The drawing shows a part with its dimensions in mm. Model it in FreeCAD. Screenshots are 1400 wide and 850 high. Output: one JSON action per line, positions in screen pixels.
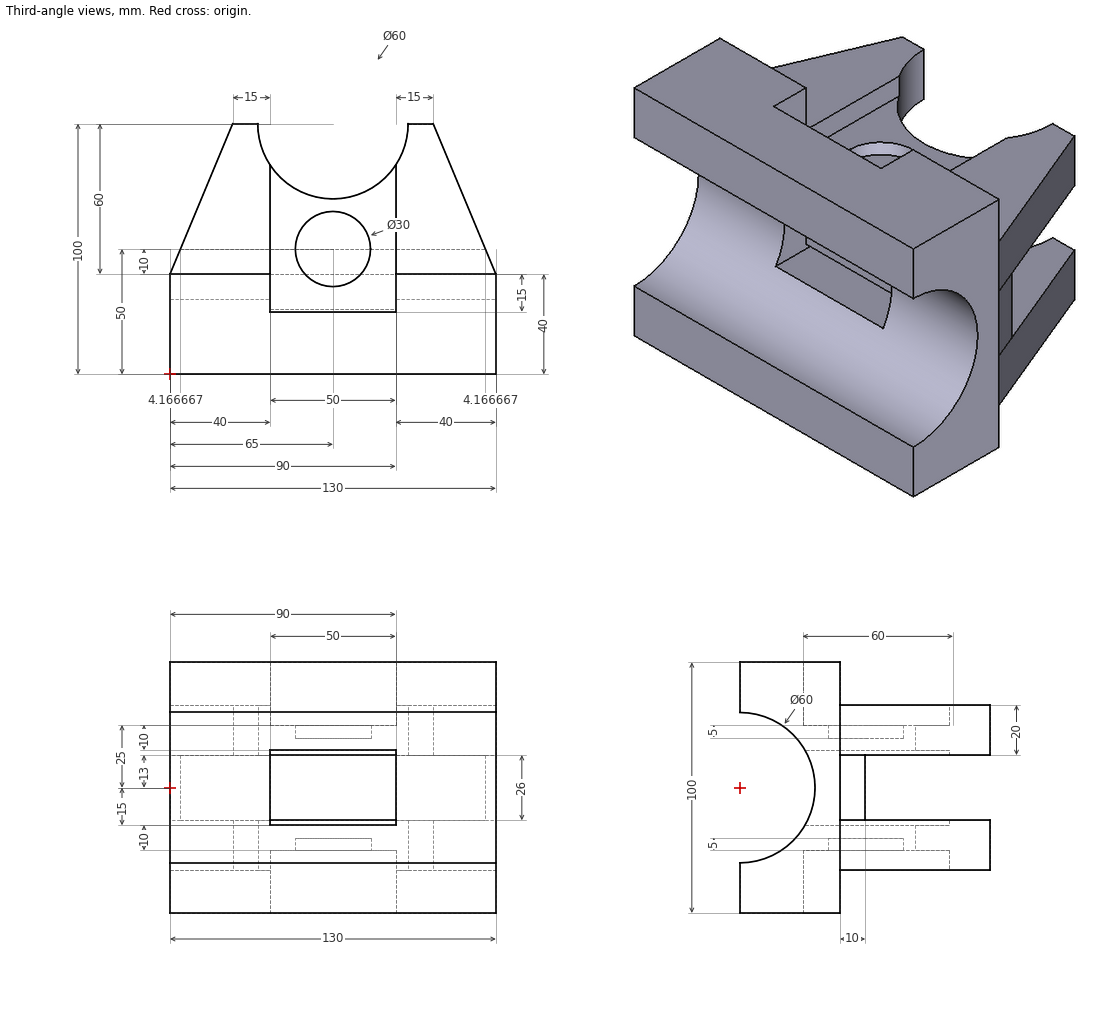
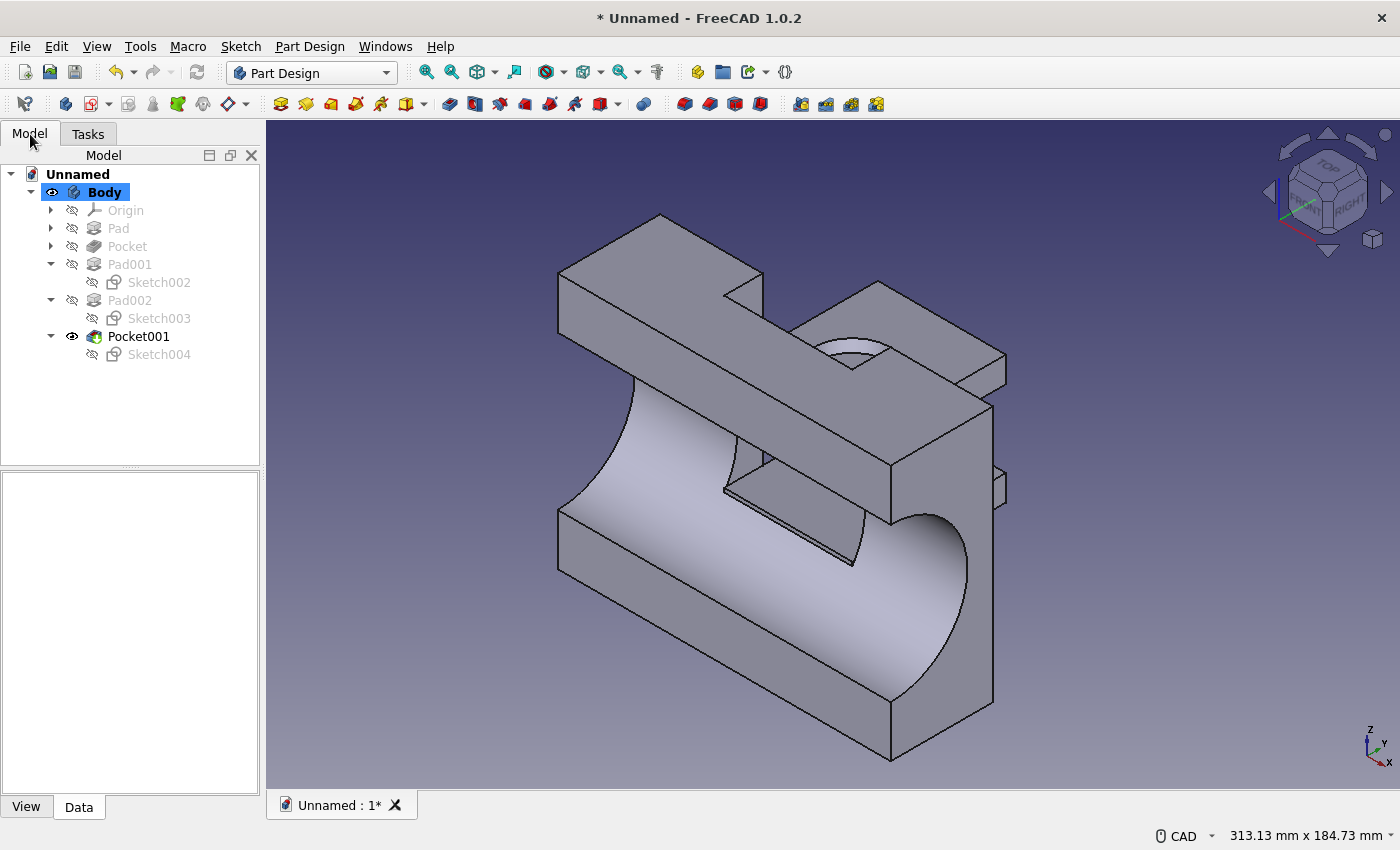
{"action": "left_click", "coordinate": [51, 210]}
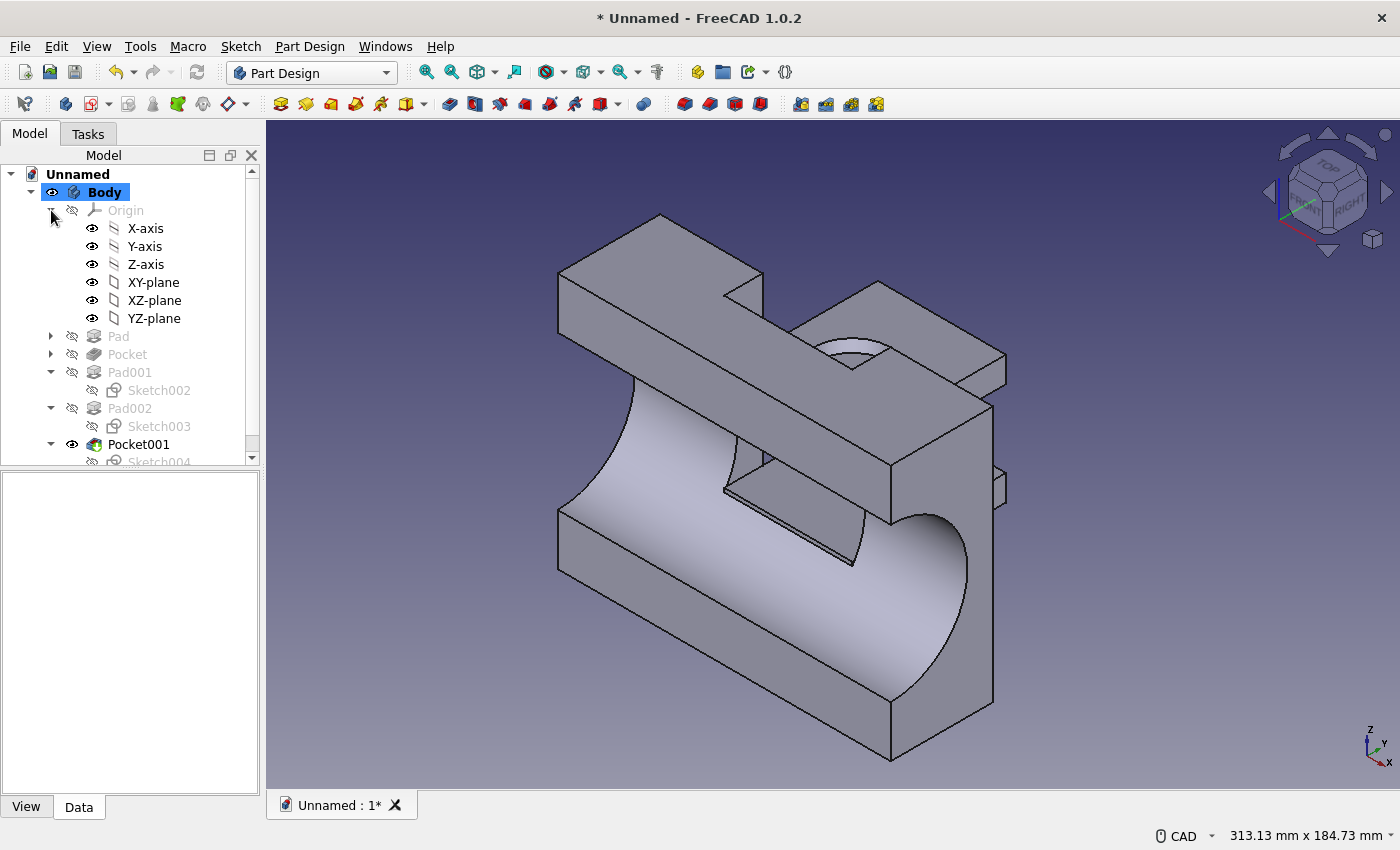
{"action": "left_click", "coordinate": [137, 282]}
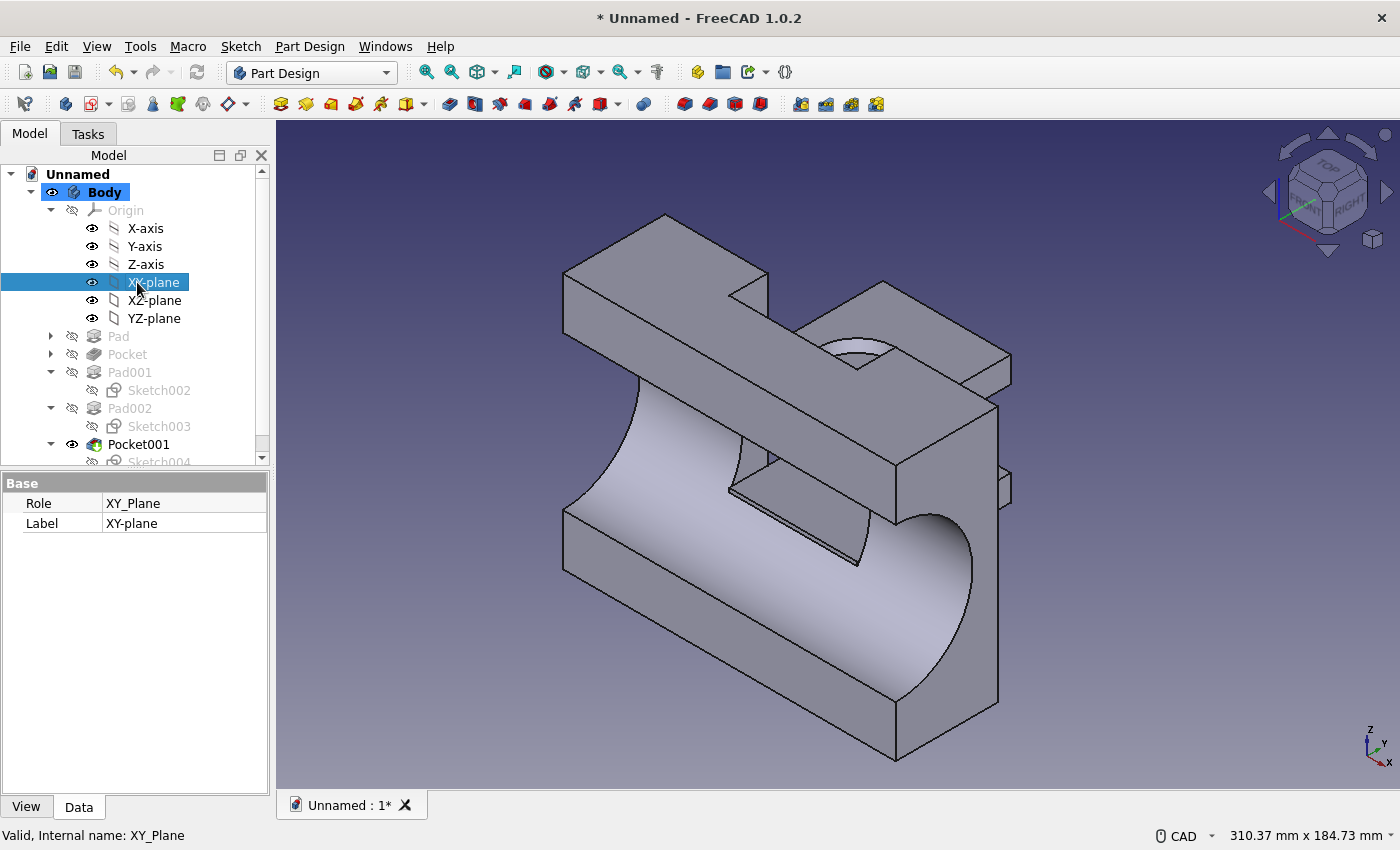
{"action": "left_click", "coordinate": [228, 104]}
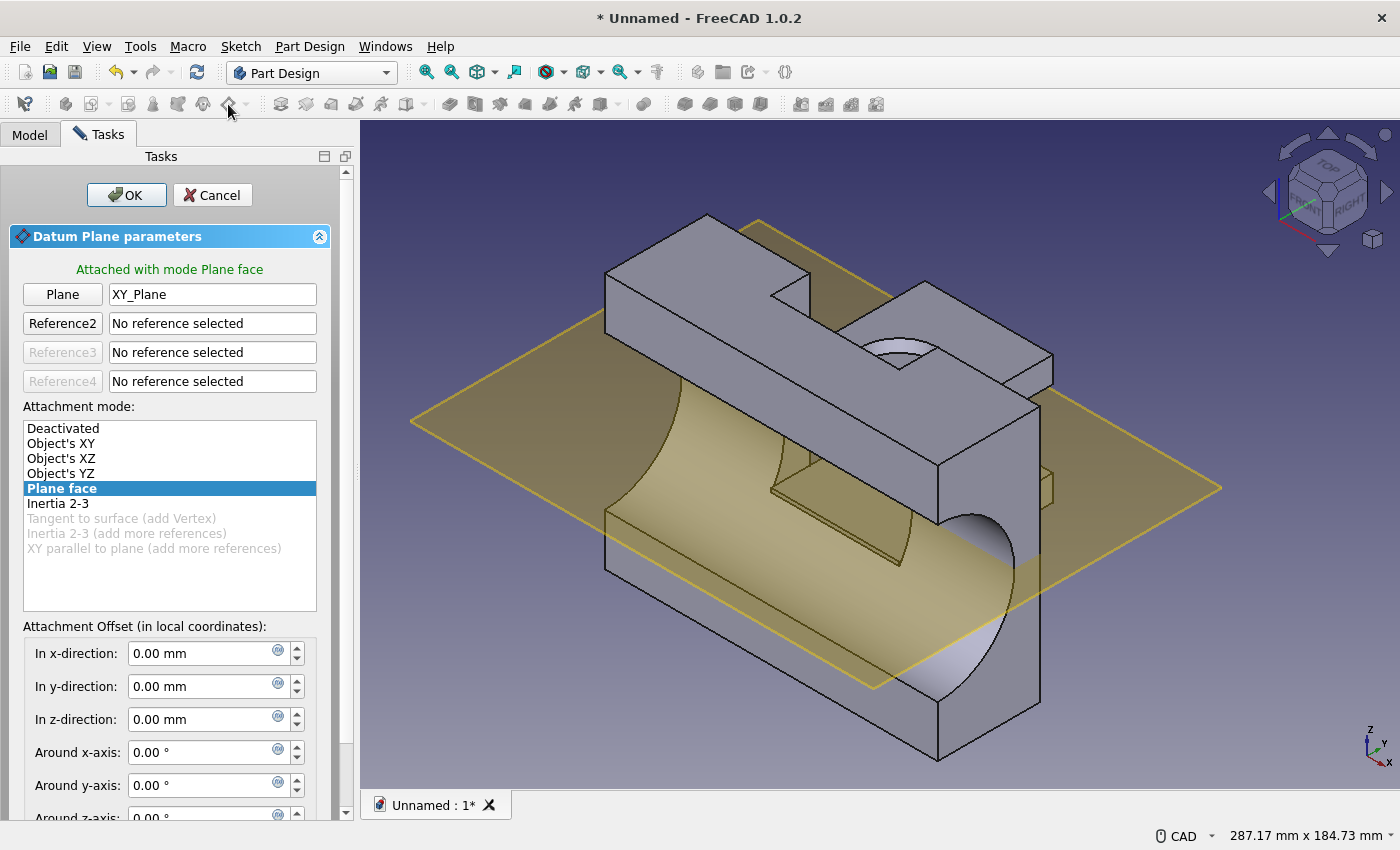
{"action": "triple_click", "coordinate": [210, 720]}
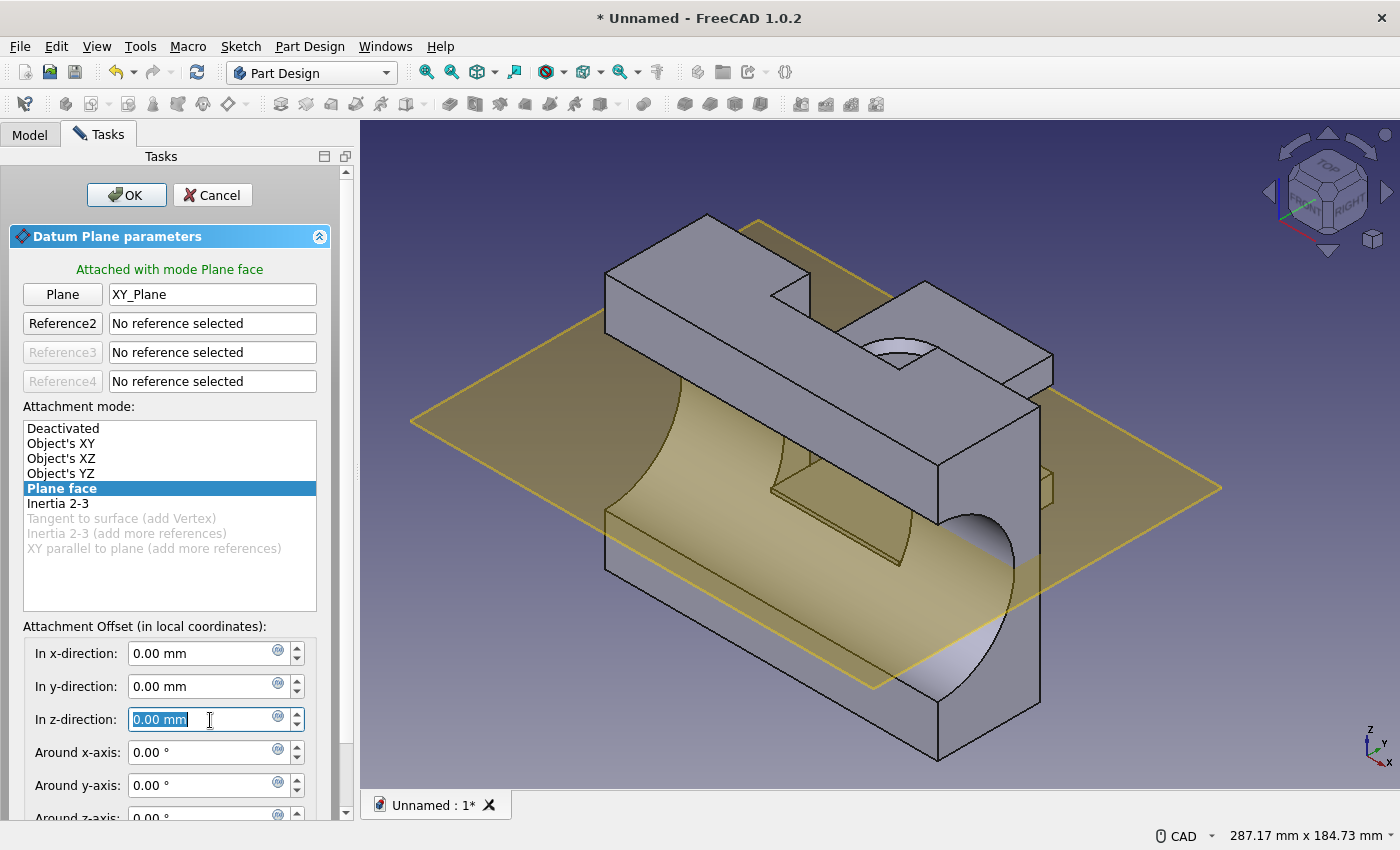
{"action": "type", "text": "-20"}
{"action": "key", "text": "Tab"}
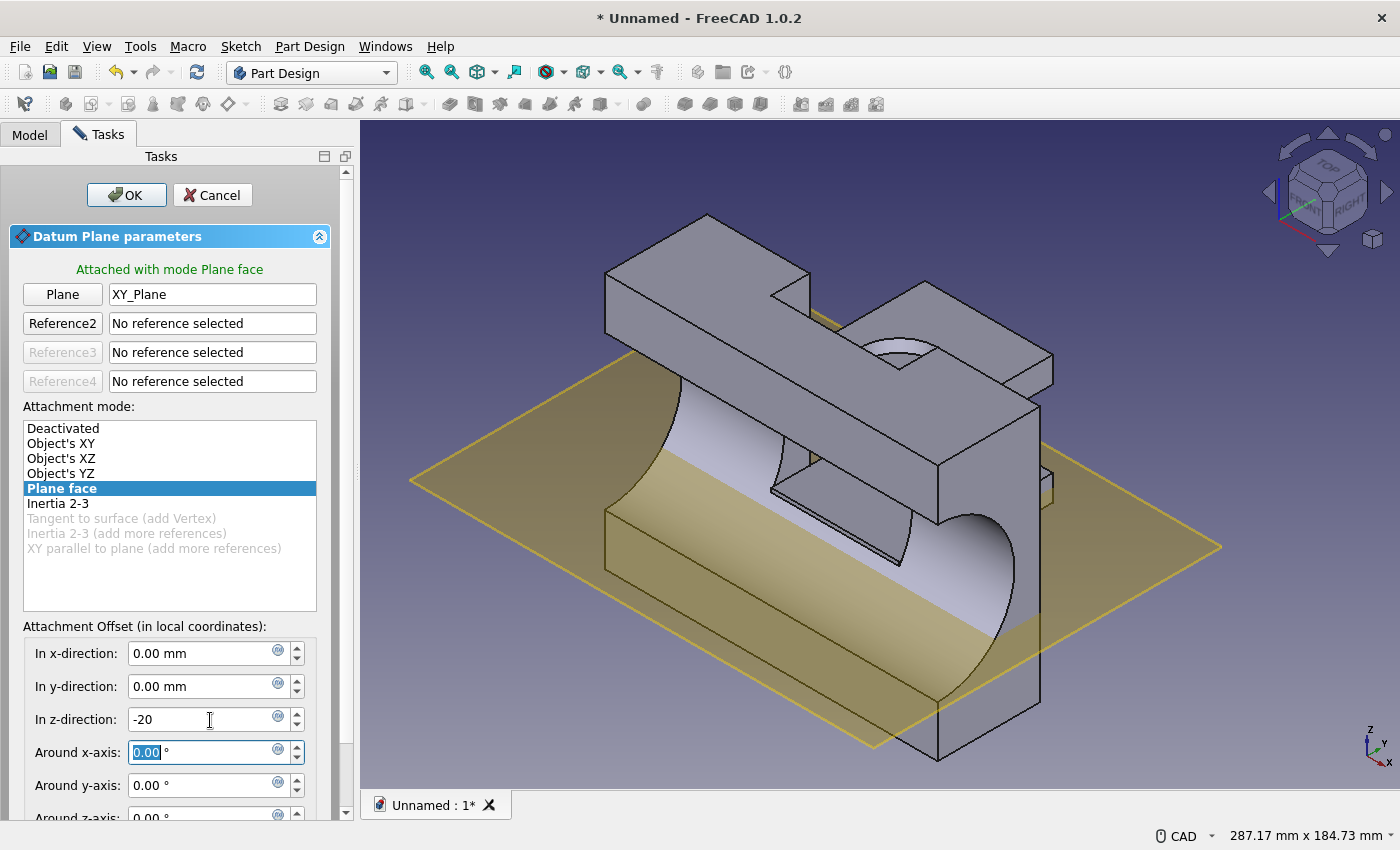
{"action": "left_click", "coordinate": [127, 195]}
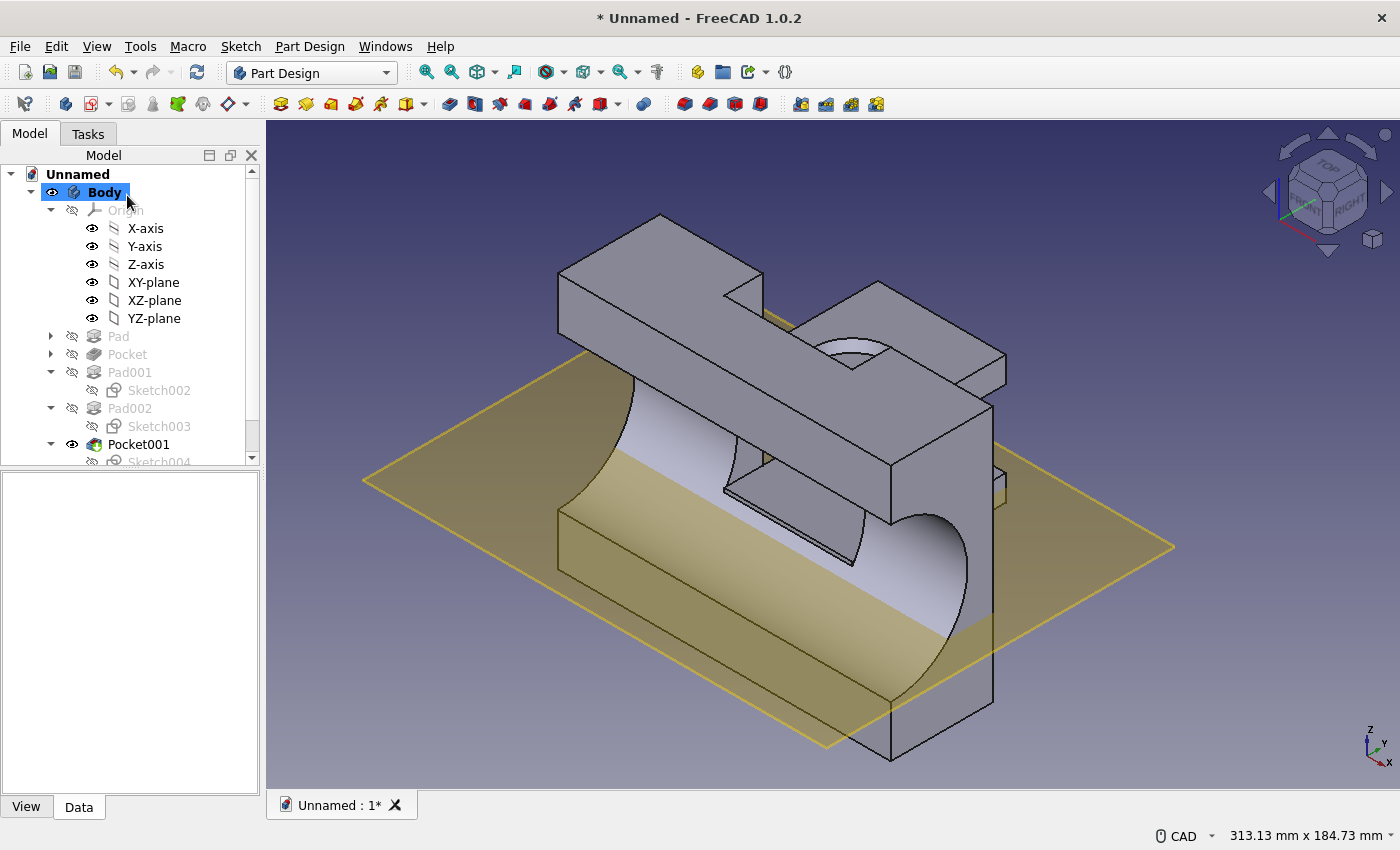
{"action": "scroll", "coordinate": [101, 314], "scroll_direction": "down", "scroll_amount": 3}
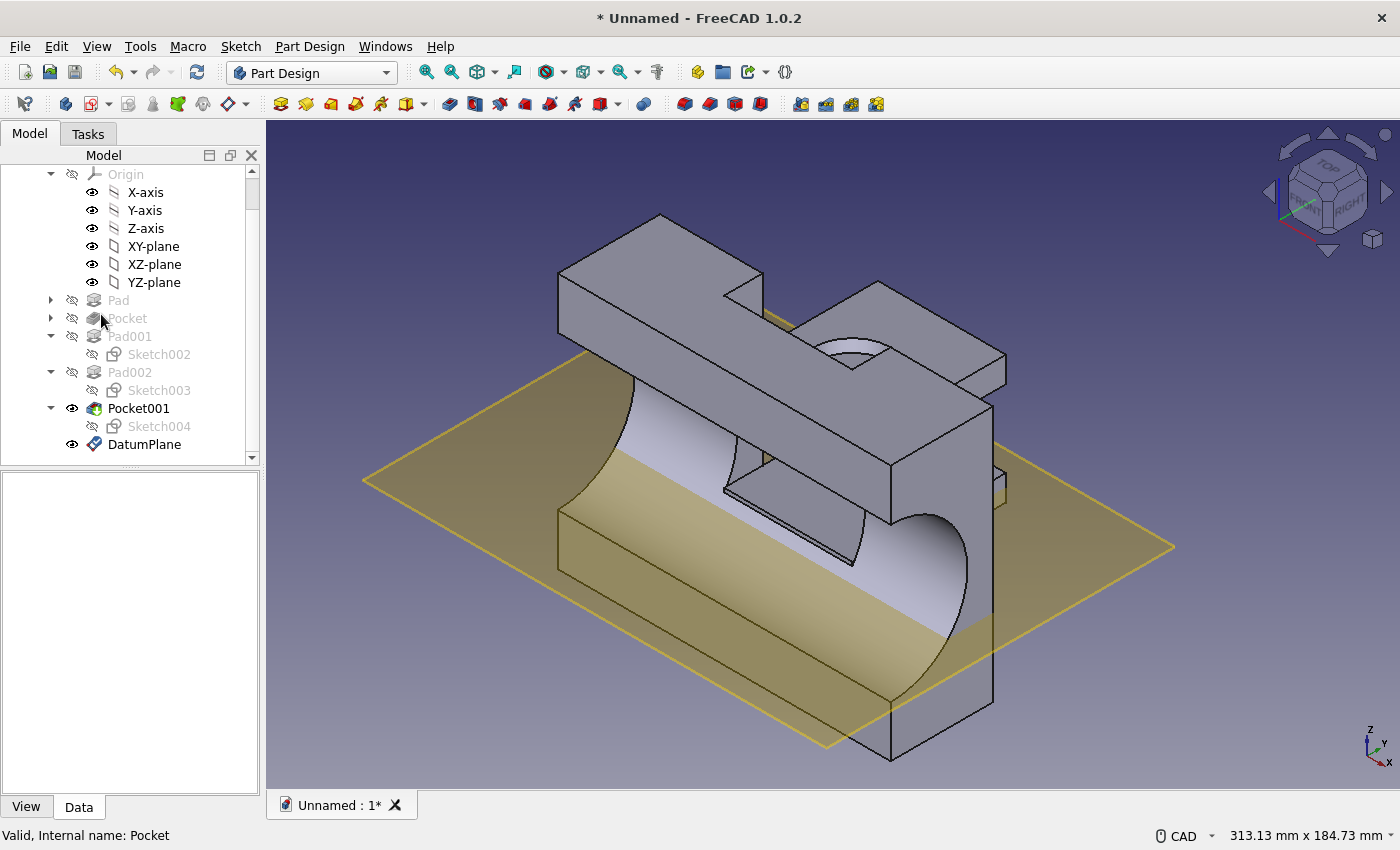
{"action": "left_click", "coordinate": [117, 444]}